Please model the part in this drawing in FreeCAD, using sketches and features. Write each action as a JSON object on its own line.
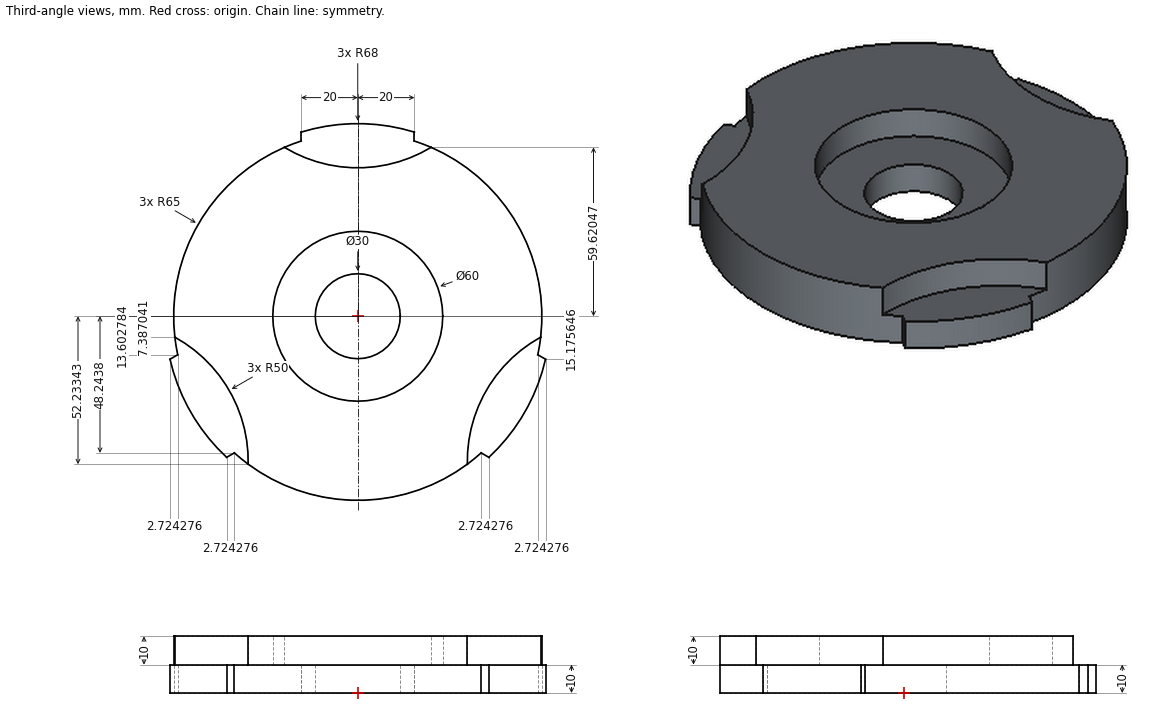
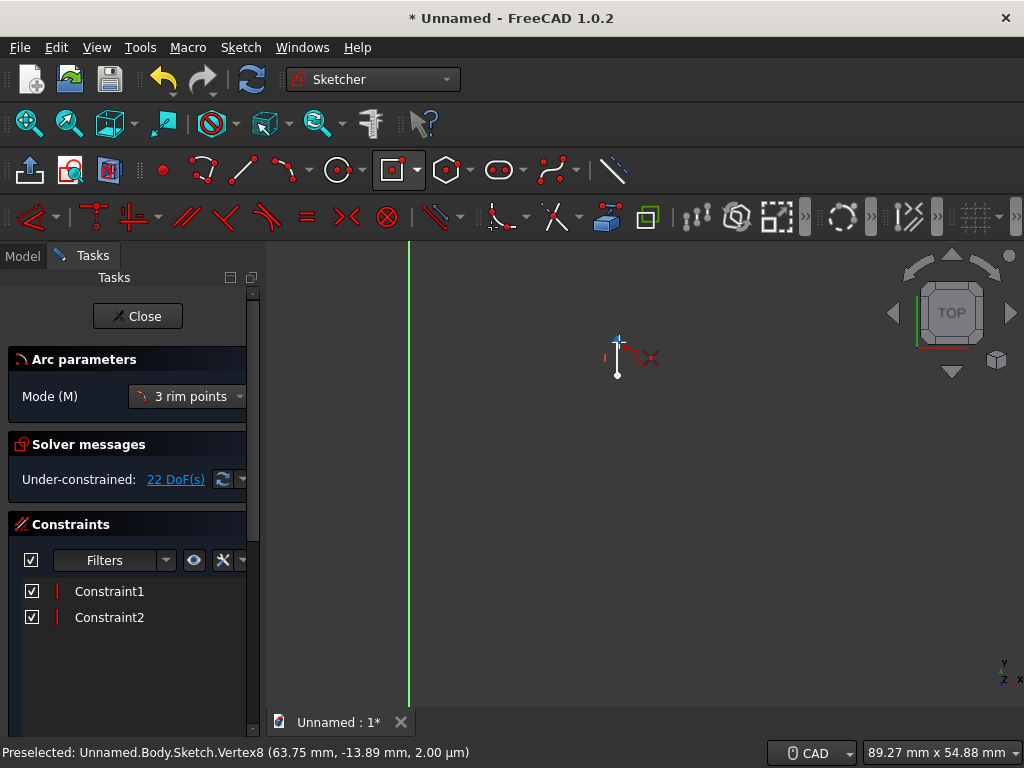
{"action": "left_click", "coordinate": [617, 340]}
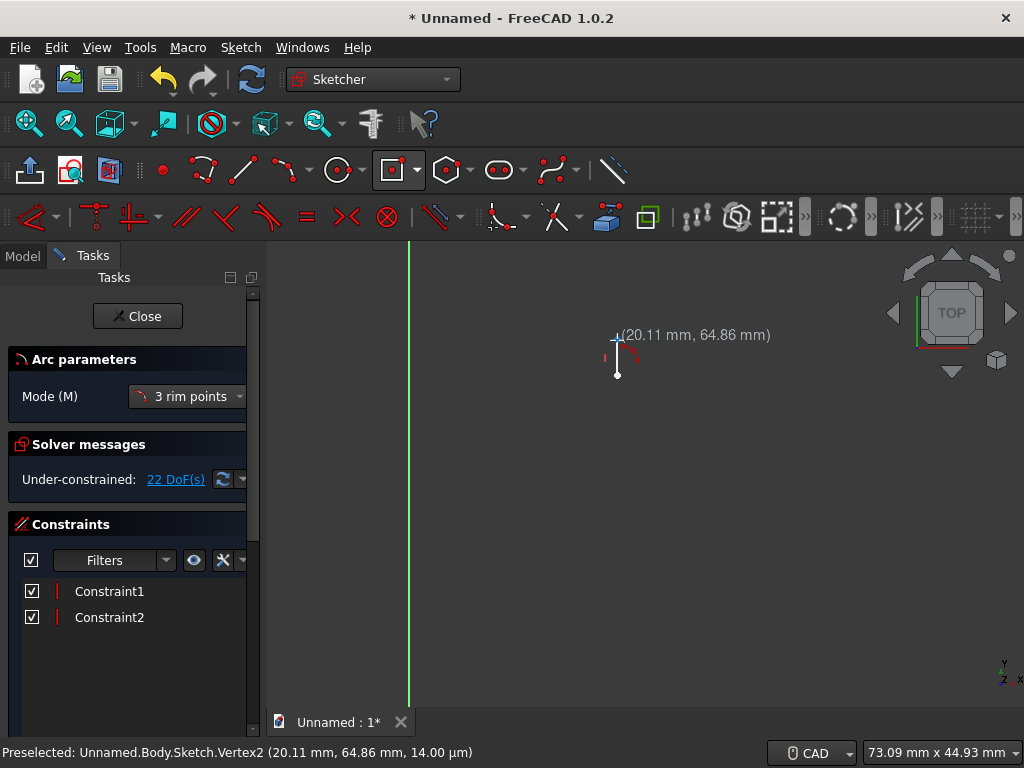
{"action": "scroll", "coordinate": [619, 342], "scroll_direction": "down", "scroll_amount": 8}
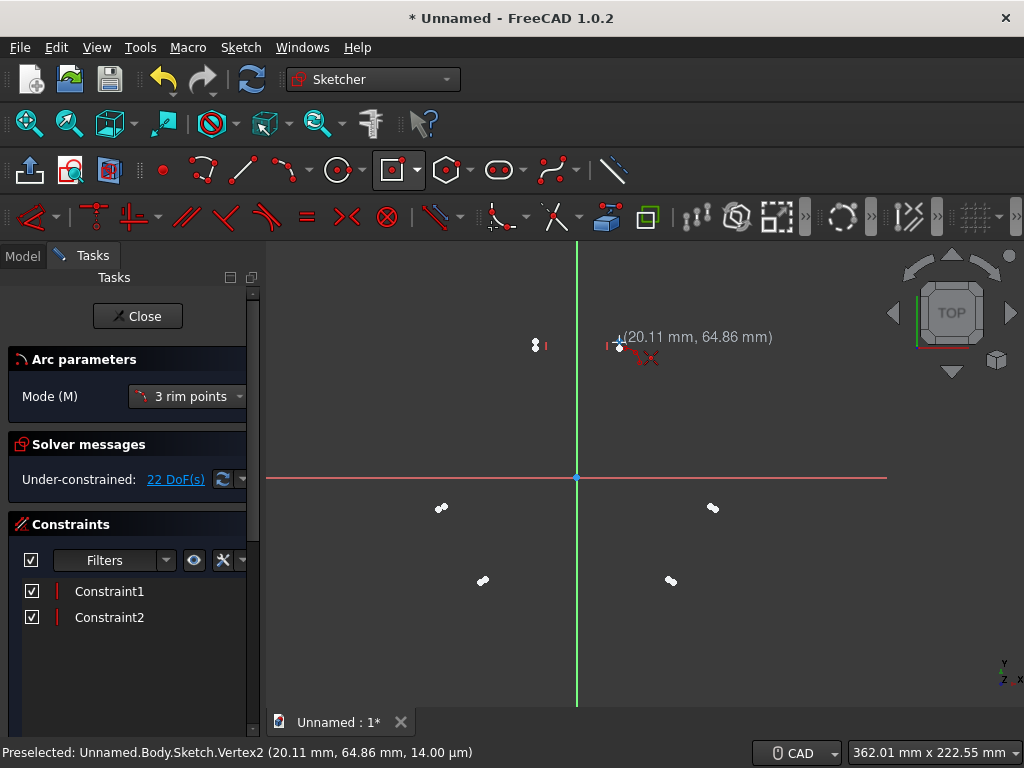
{"action": "scroll", "coordinate": [535, 342], "scroll_direction": "up", "scroll_amount": 8}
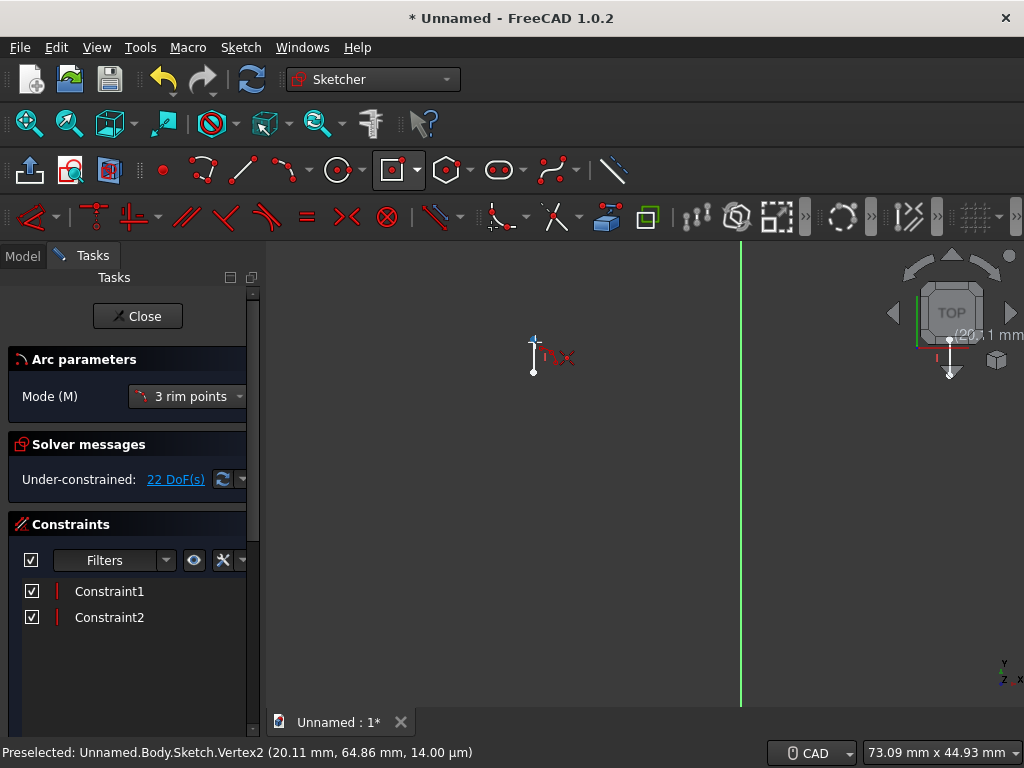
{"action": "left_click", "coordinate": [534, 340]}
{"action": "left_click", "coordinate": [783, 309]}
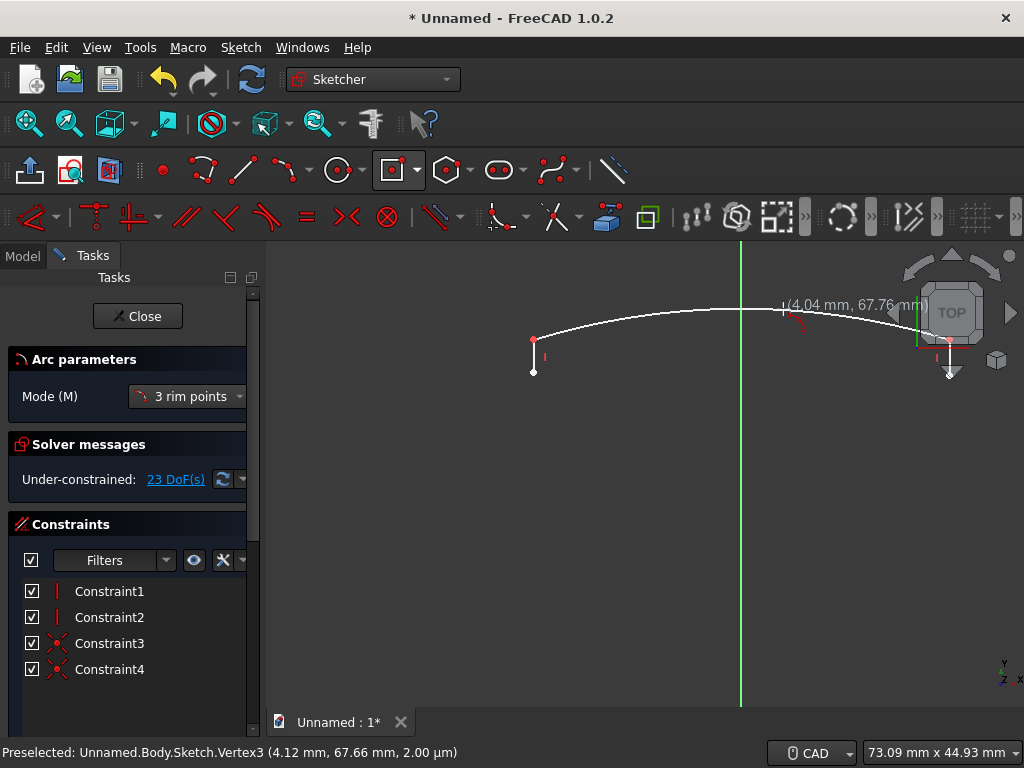
{"action": "left_click", "coordinate": [534, 373]}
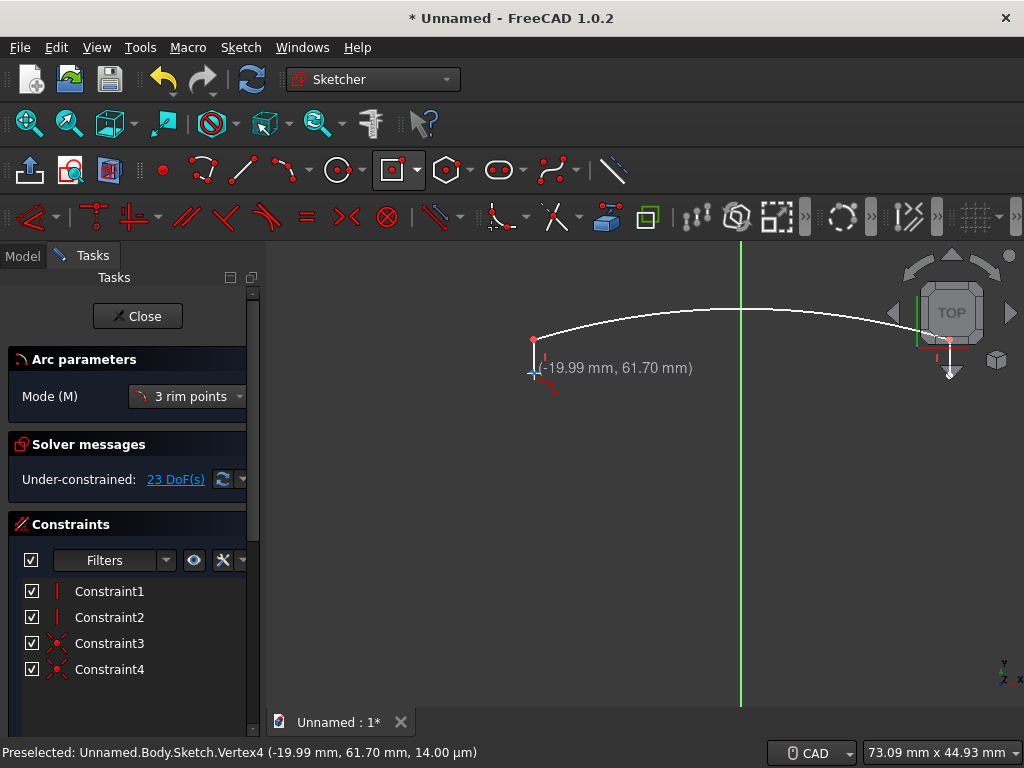
{"action": "scroll", "coordinate": [535, 342], "scroll_direction": "down", "scroll_amount": 8}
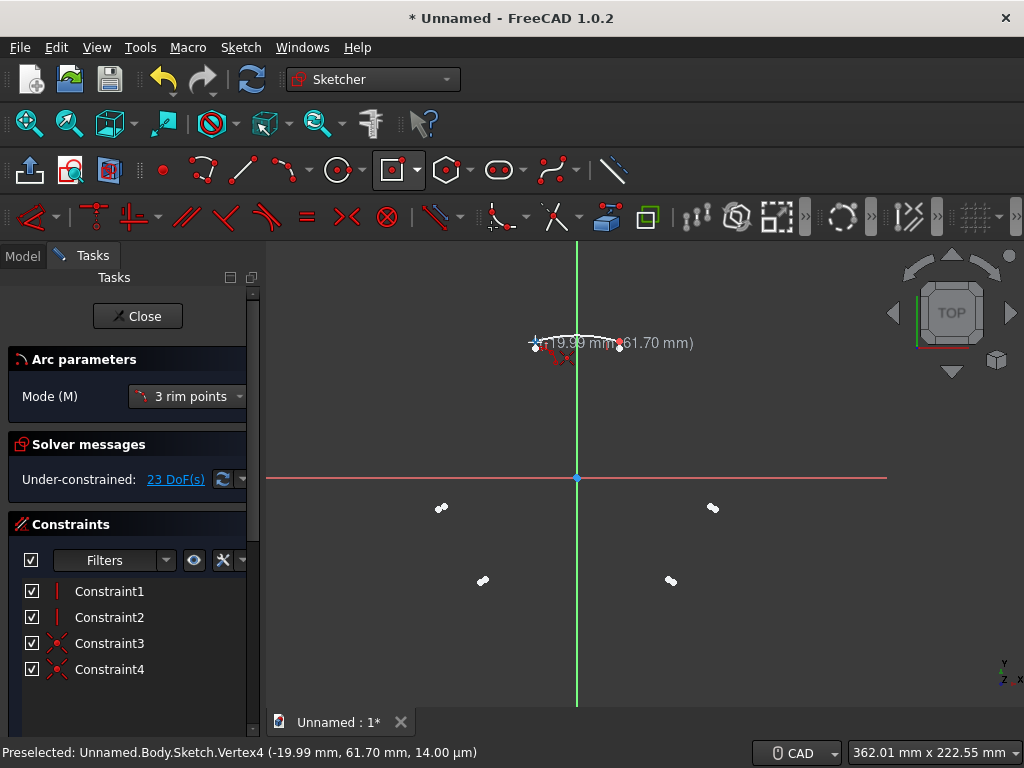
{"action": "scroll", "coordinate": [444, 506], "scroll_direction": "up", "scroll_amount": 8}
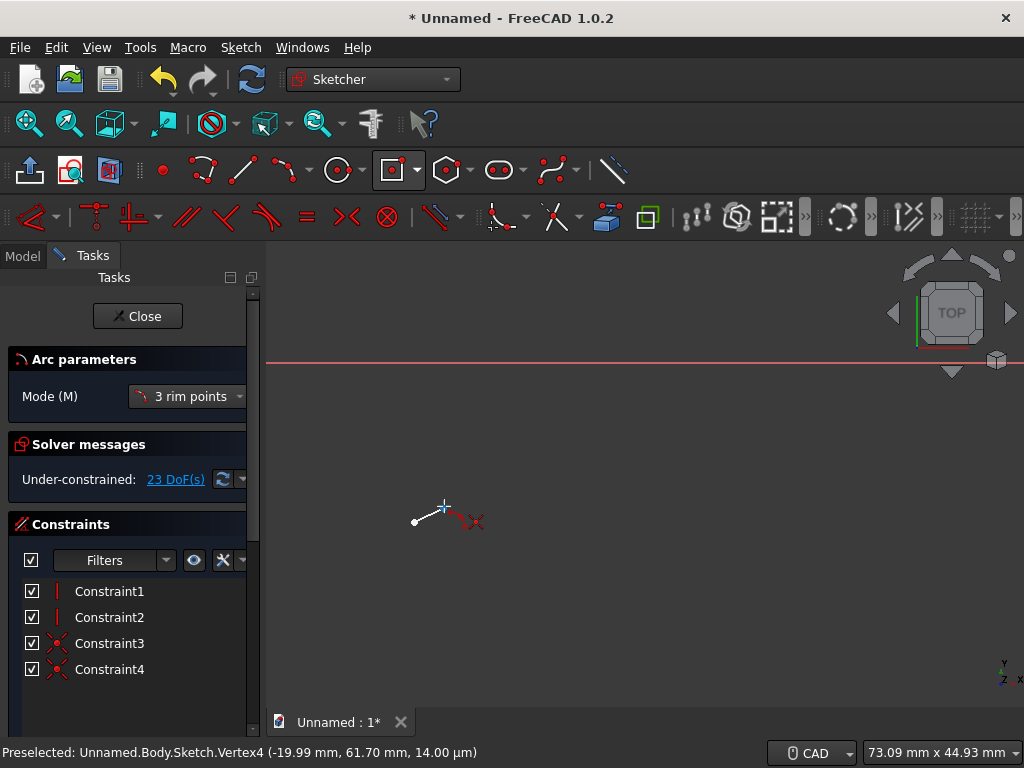
{"action": "left_click", "coordinate": [443, 509]}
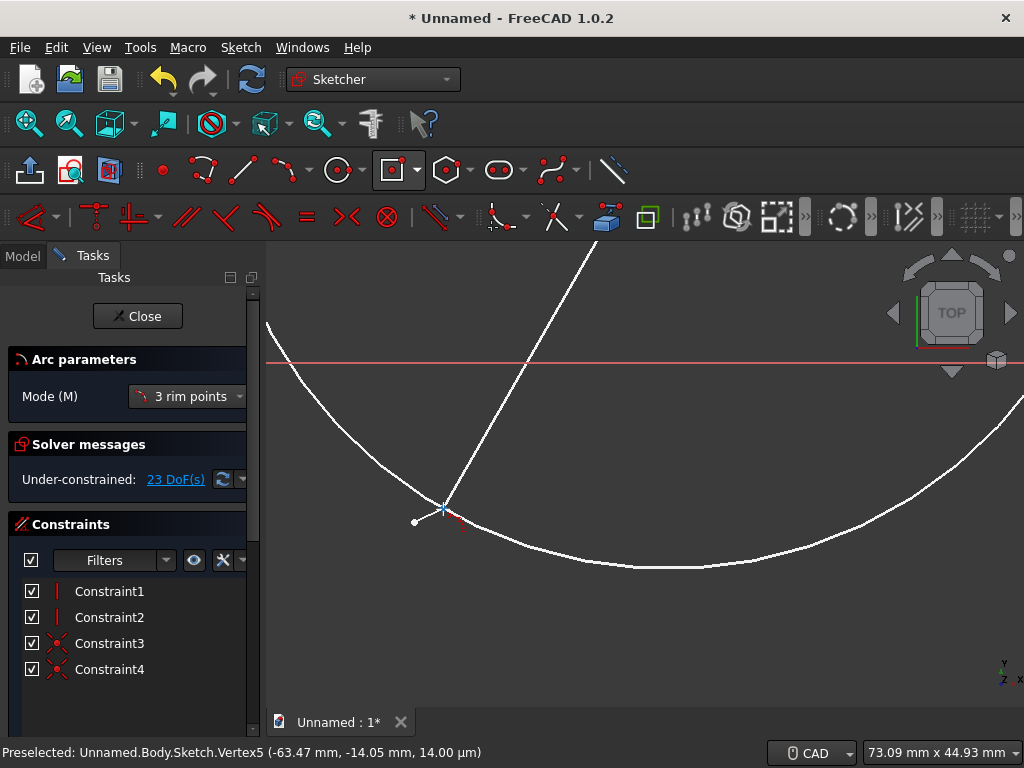
{"action": "scroll", "coordinate": [444, 506], "scroll_direction": "down", "scroll_amount": 8}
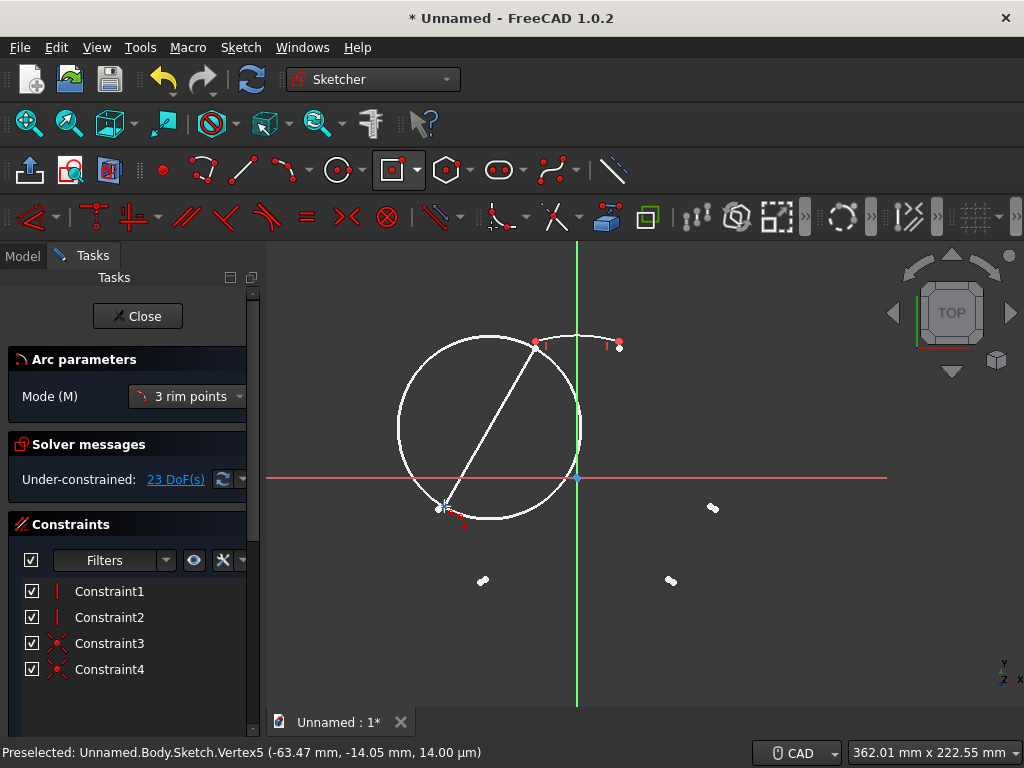
{"action": "left_click", "coordinate": [459, 410]}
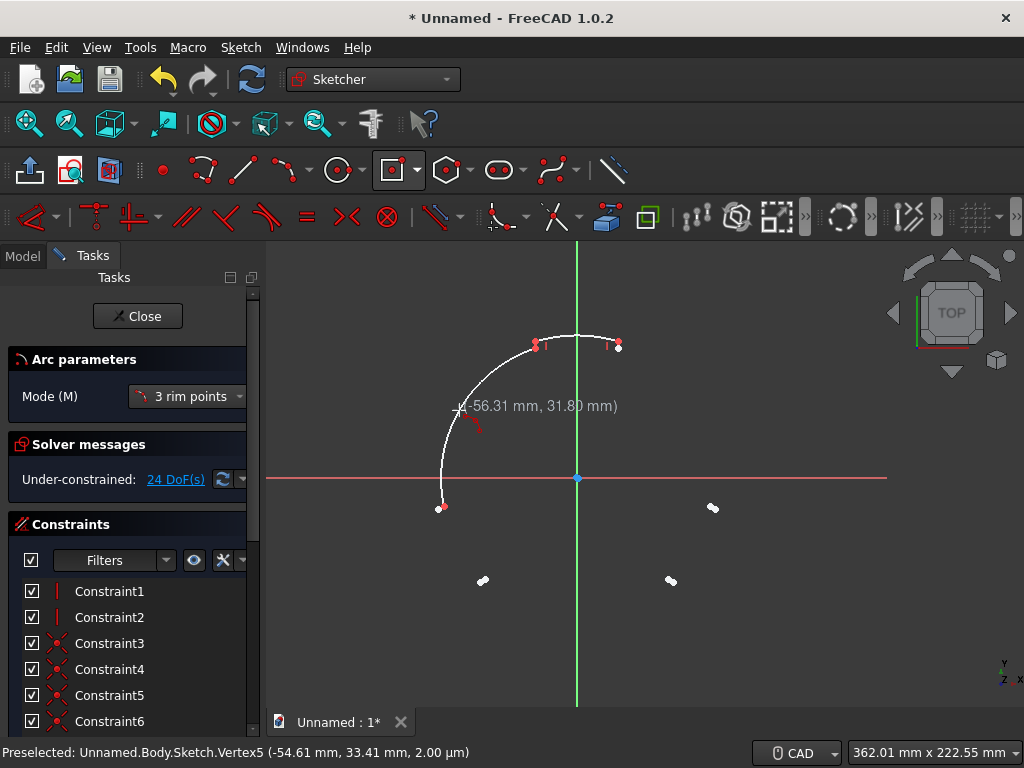
{"action": "scroll", "coordinate": [438, 509], "scroll_direction": "up", "scroll_amount": 8}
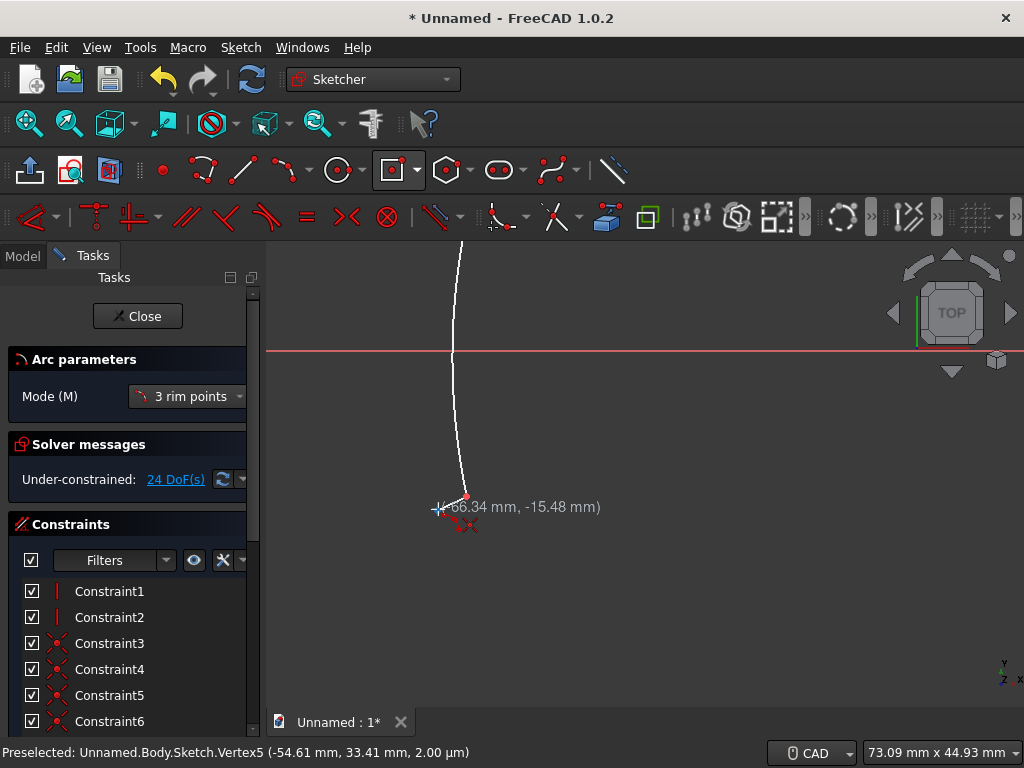
{"action": "left_click", "coordinate": [438, 510]}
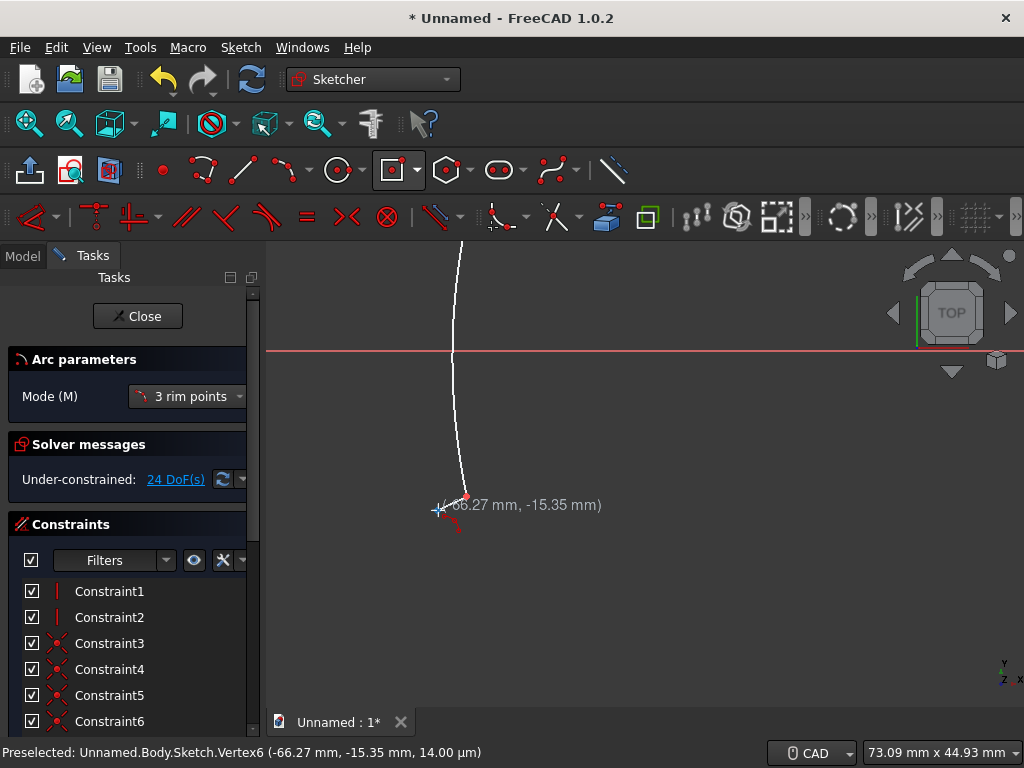
{"action": "scroll", "coordinate": [438, 509], "scroll_direction": "down", "scroll_amount": 8}